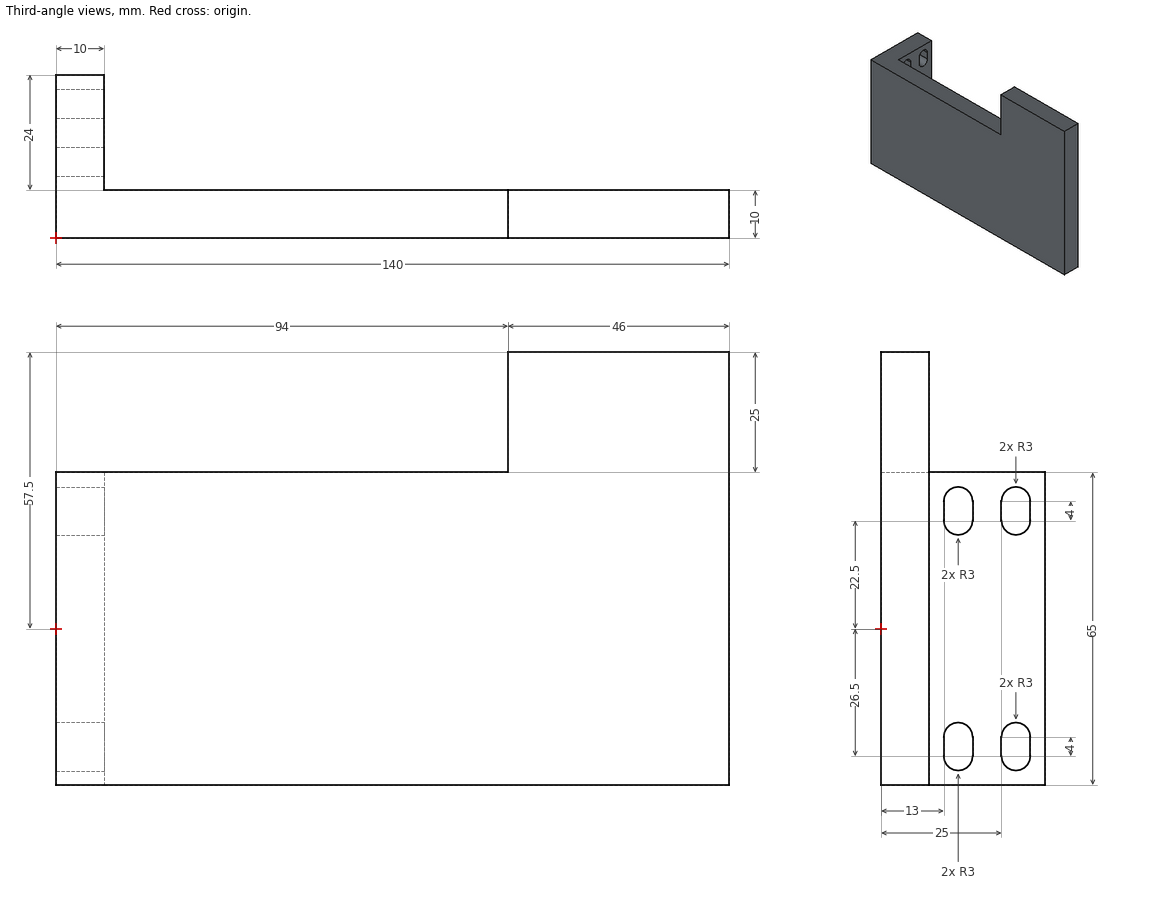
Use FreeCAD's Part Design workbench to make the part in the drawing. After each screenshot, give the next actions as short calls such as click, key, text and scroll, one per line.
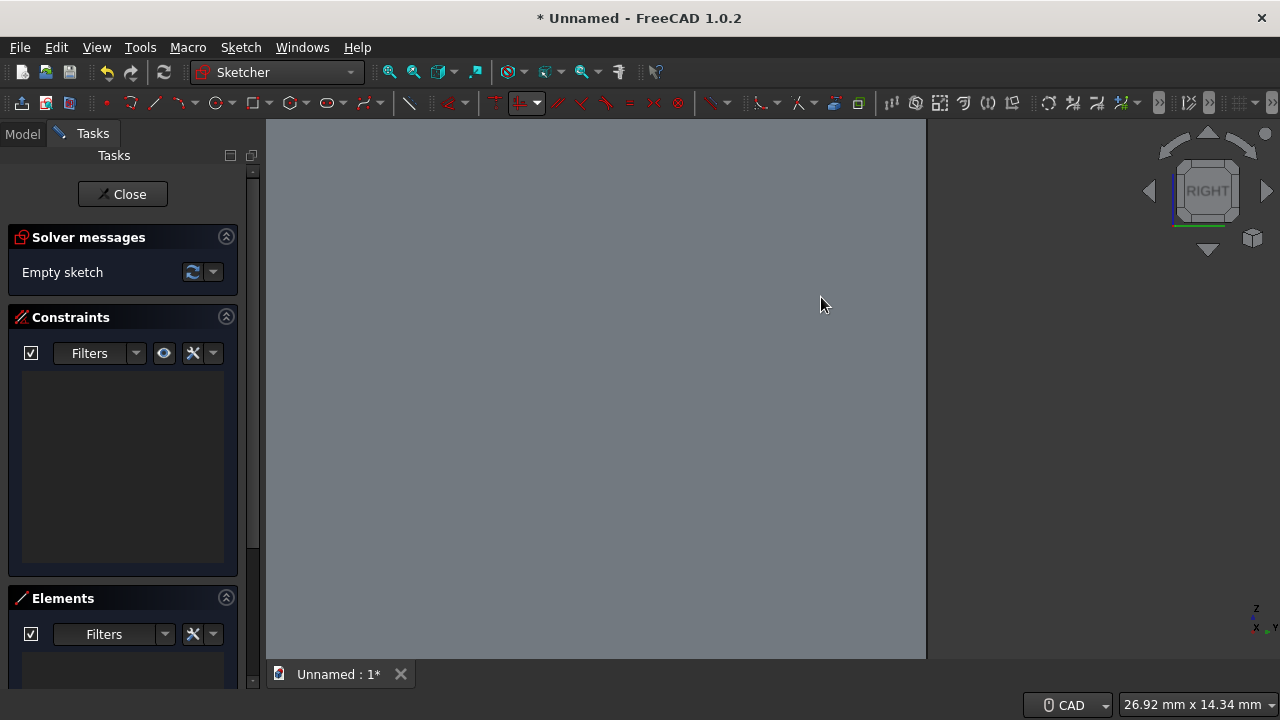
click(328, 104)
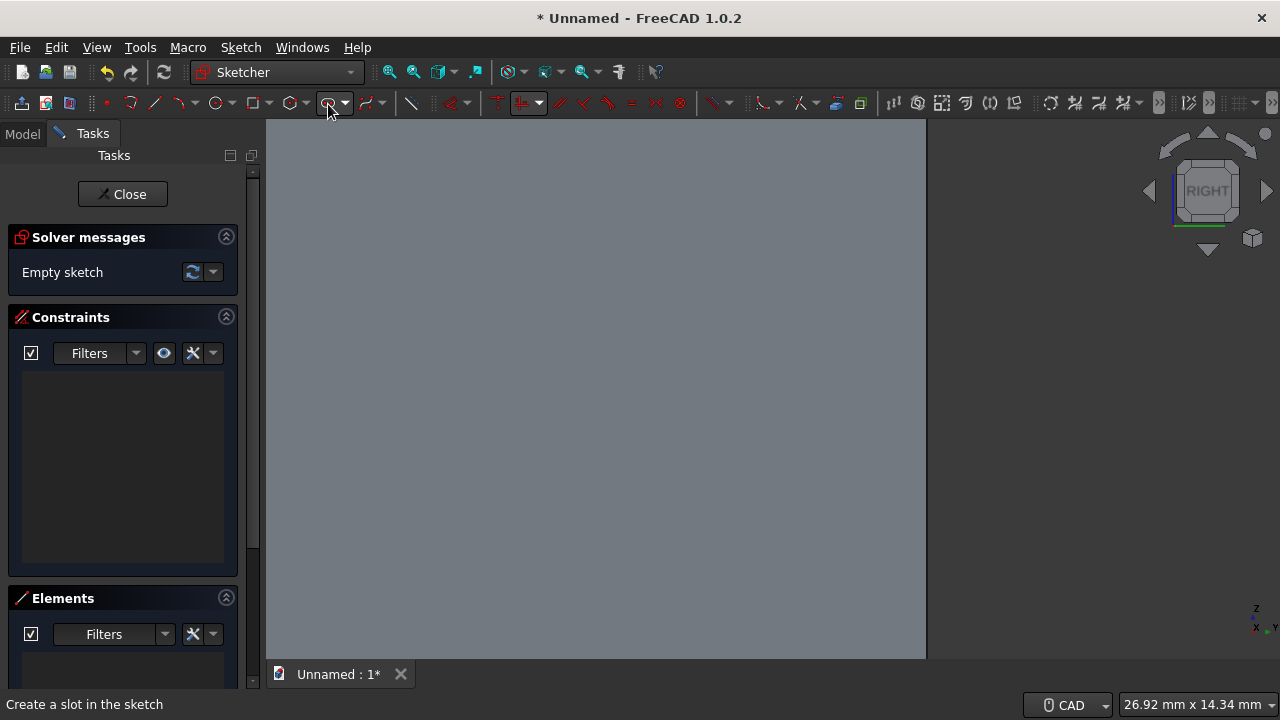
click(701, 460)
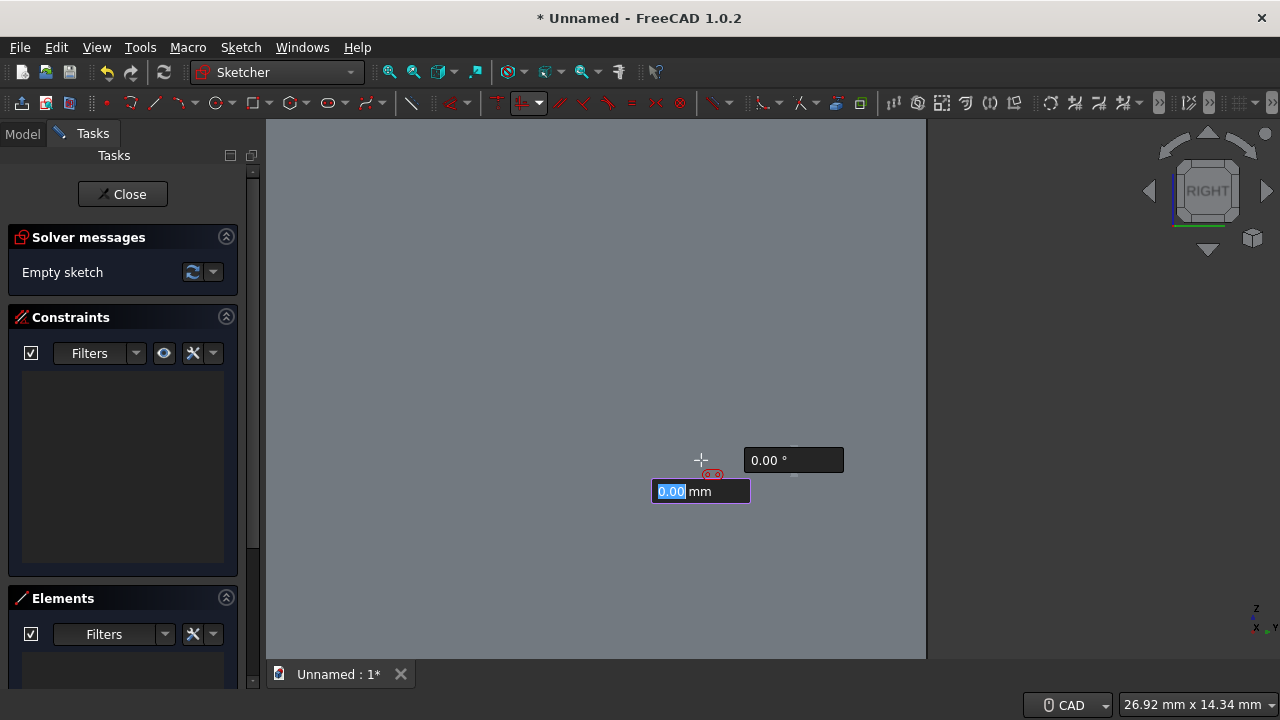
click(701, 310)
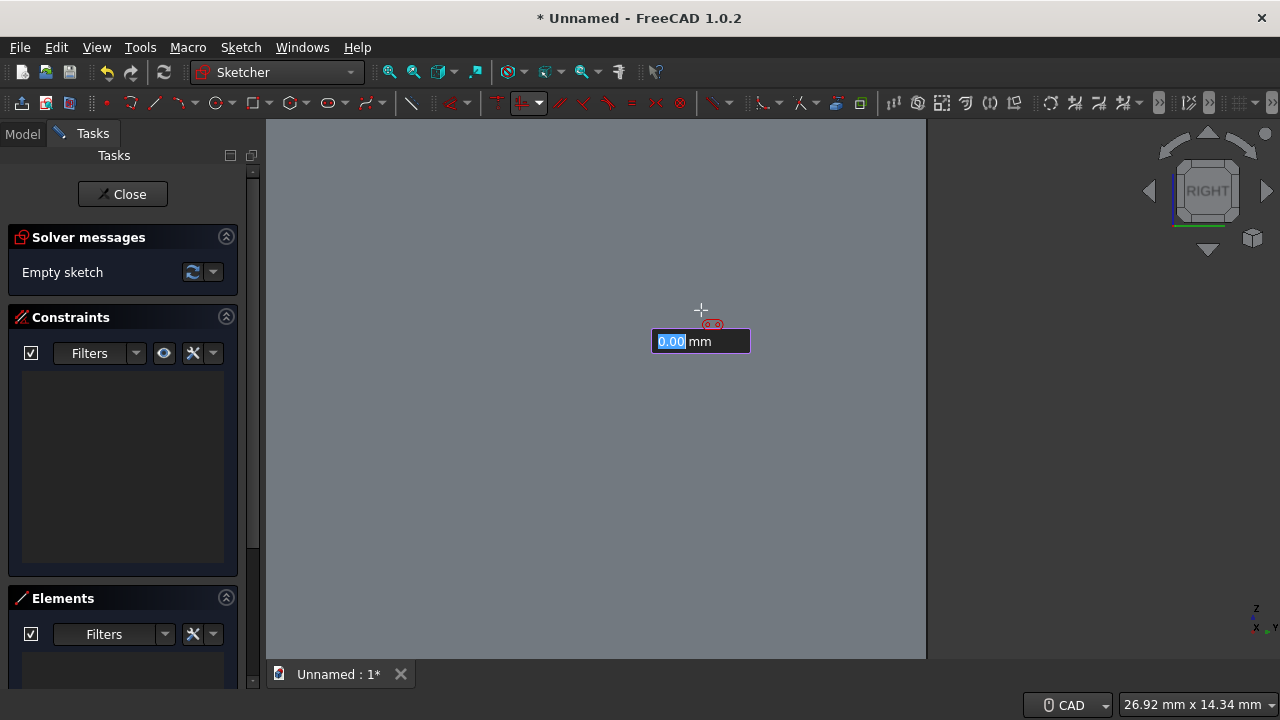
click(814, 385)
key(Escape)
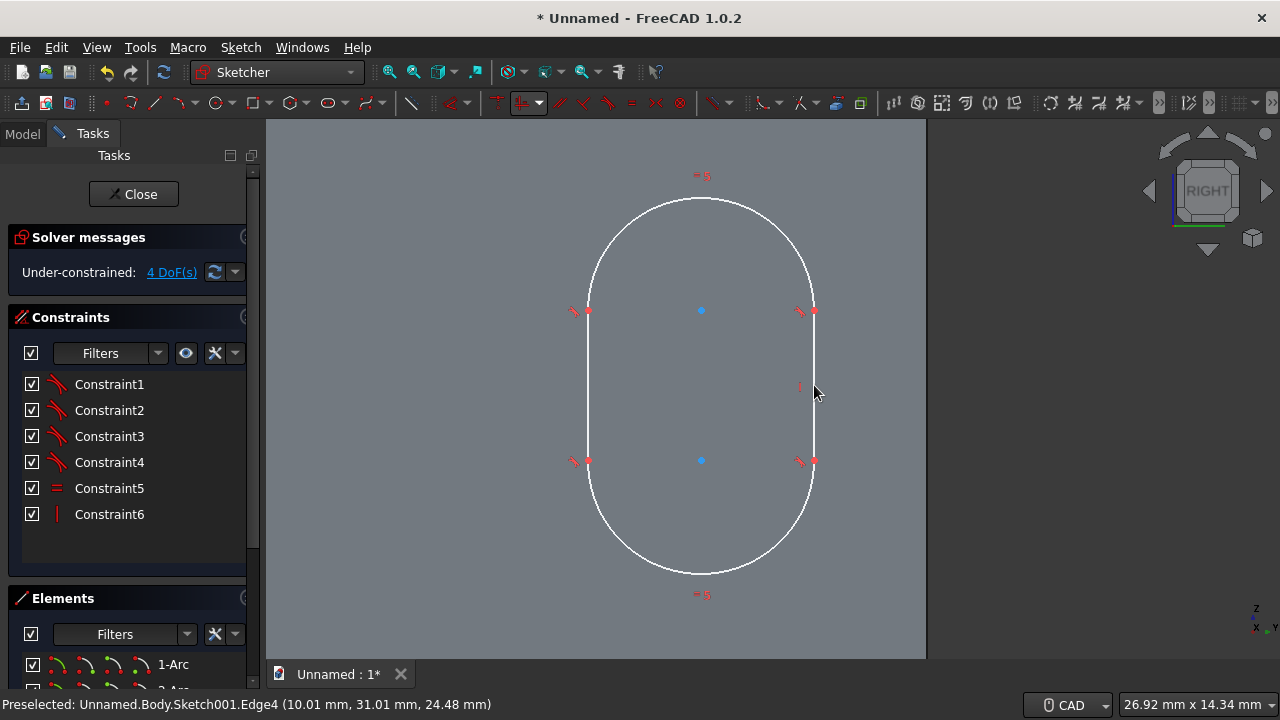
key(d)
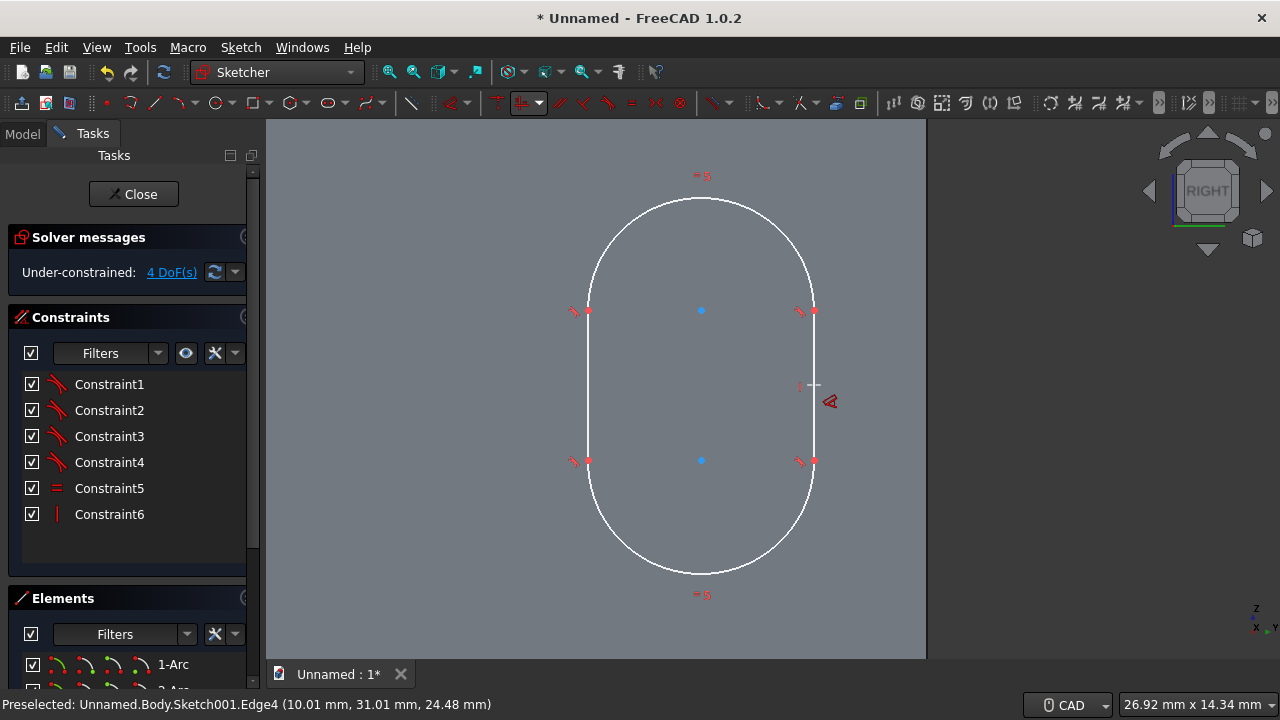
click(635, 552)
click(616, 578)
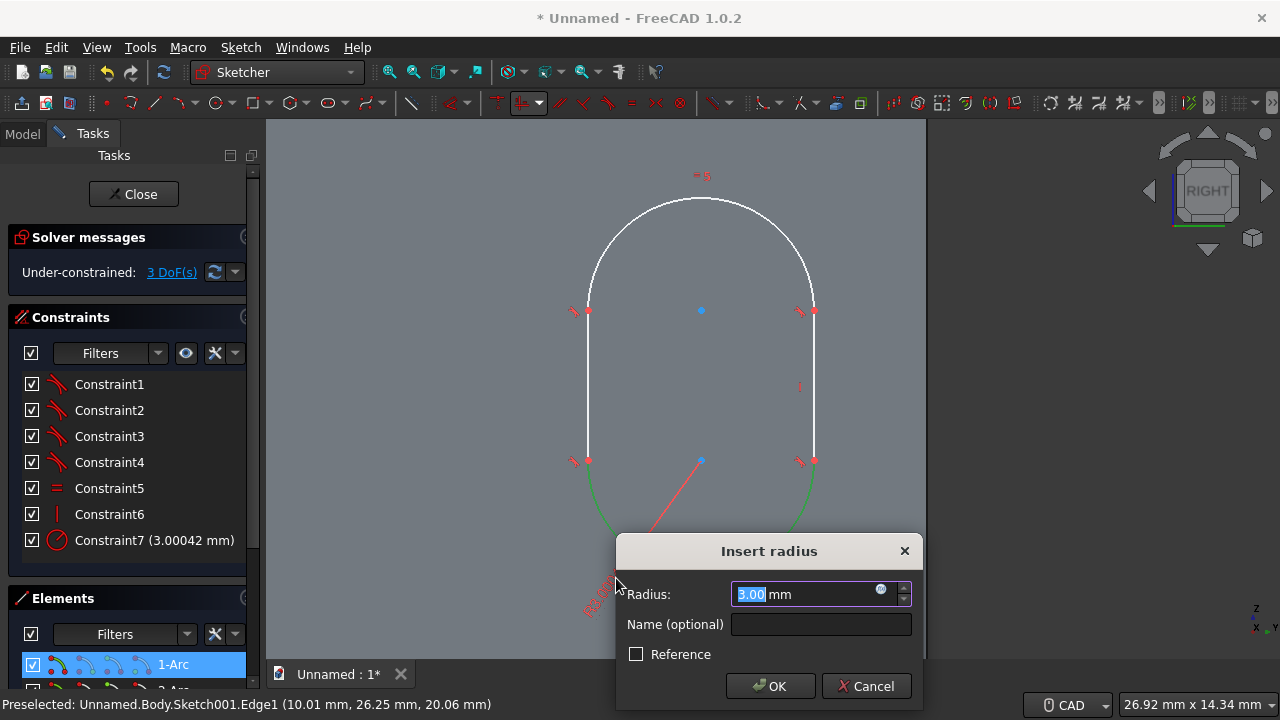
text(3)
key(Return)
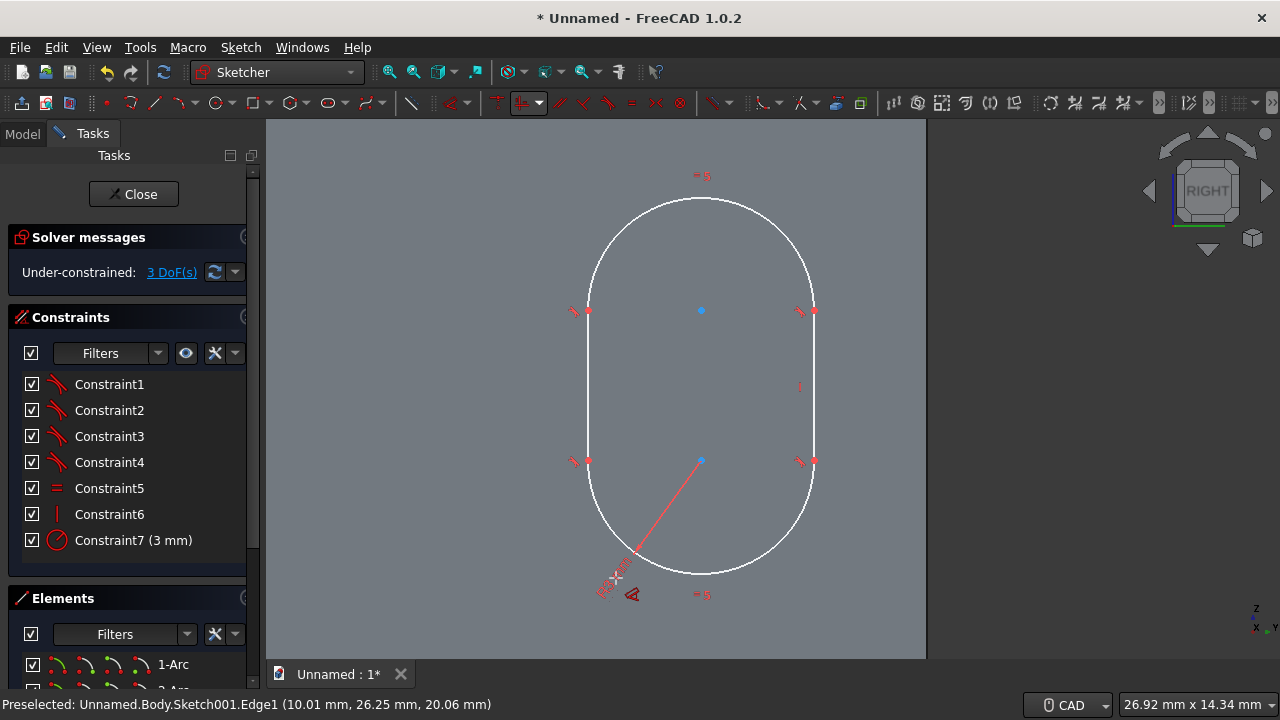
click(588, 416)
click(554, 386)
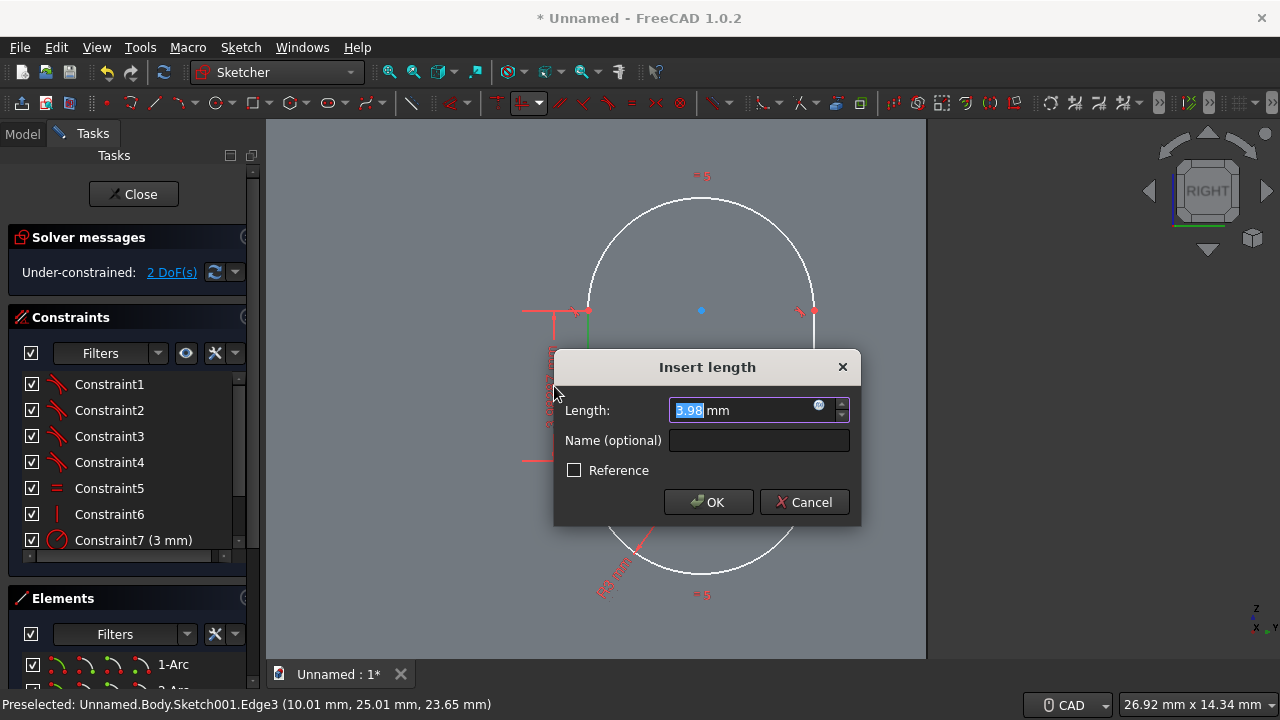
text(4)
key(Return)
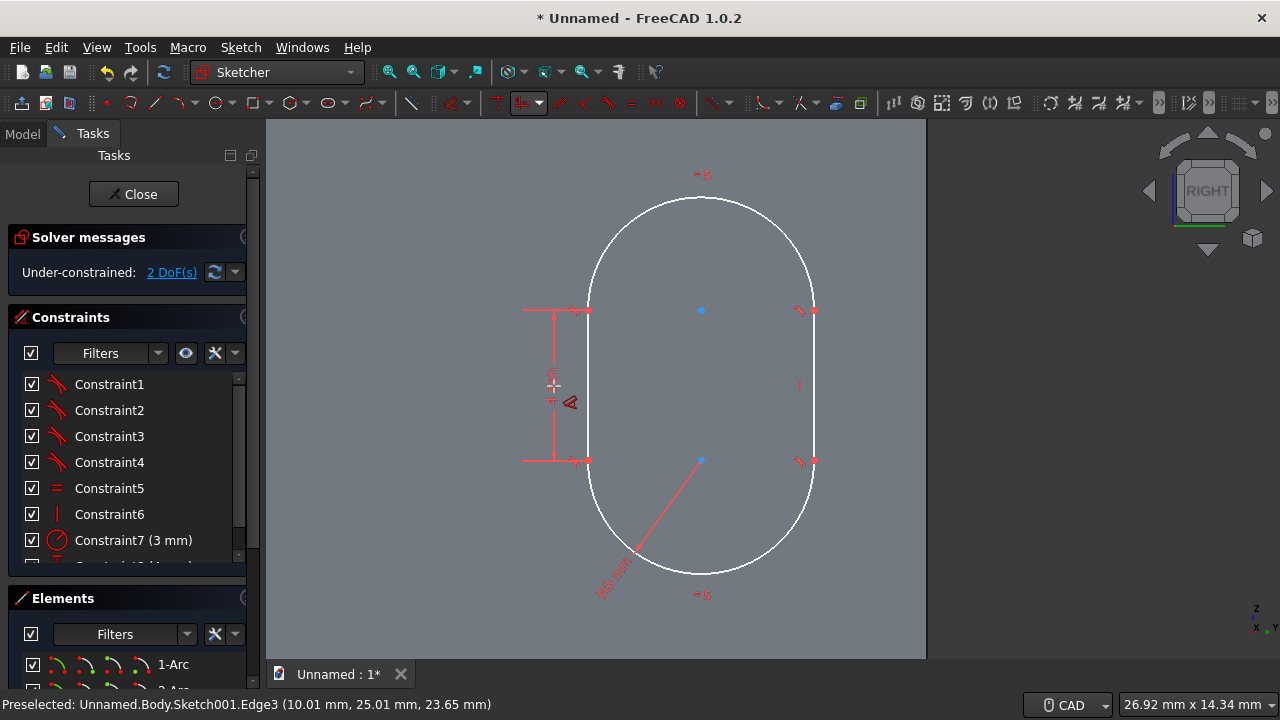
click(588, 461)
click(441, 427)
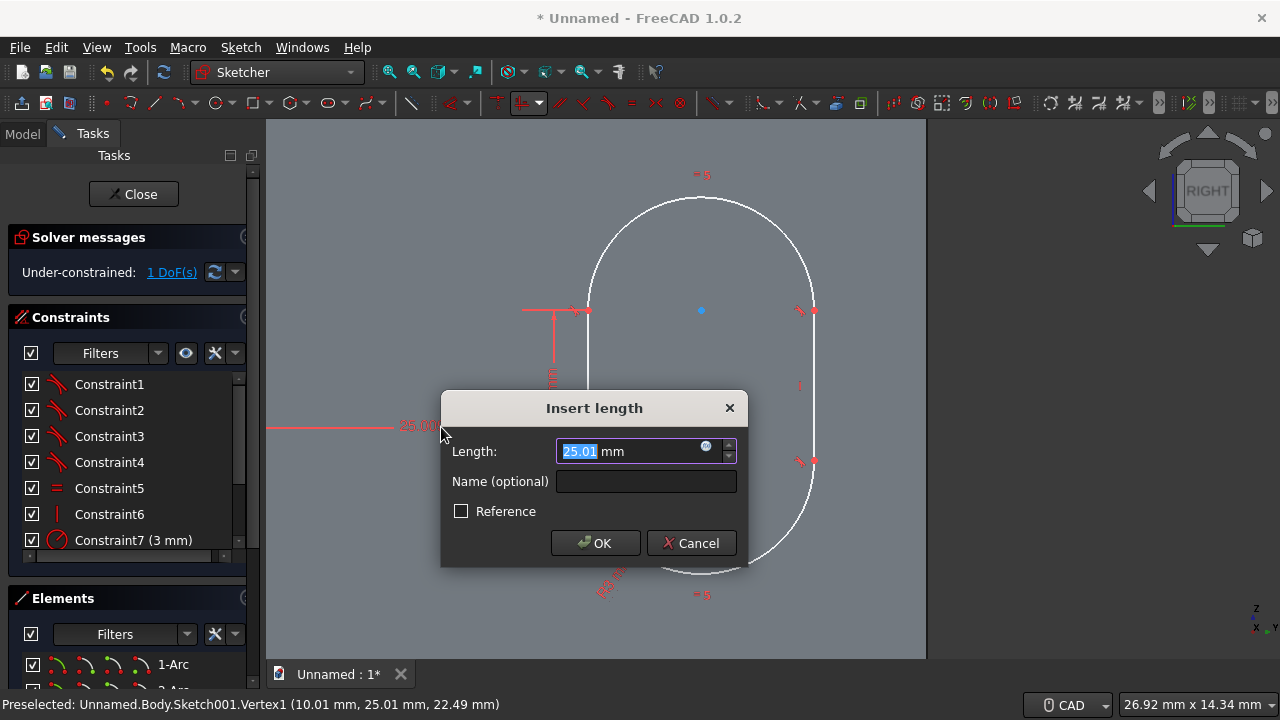
text(25)
key(Return)